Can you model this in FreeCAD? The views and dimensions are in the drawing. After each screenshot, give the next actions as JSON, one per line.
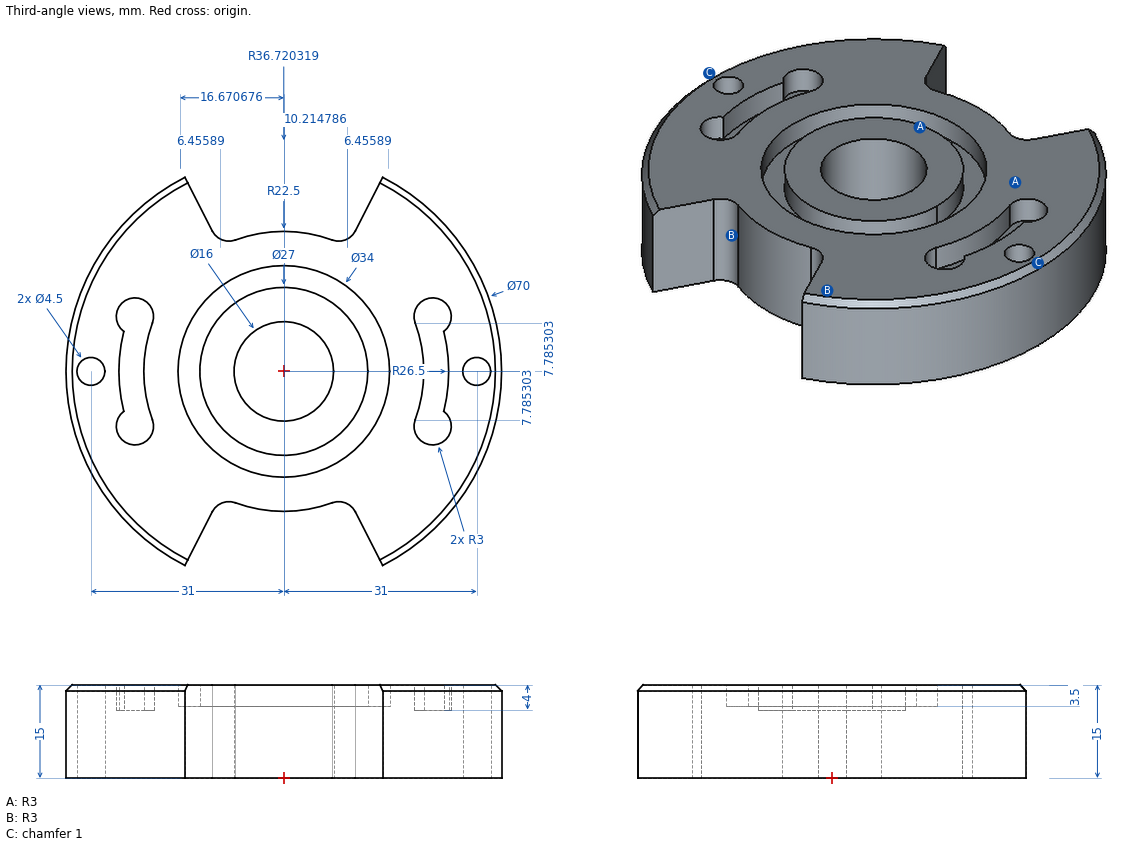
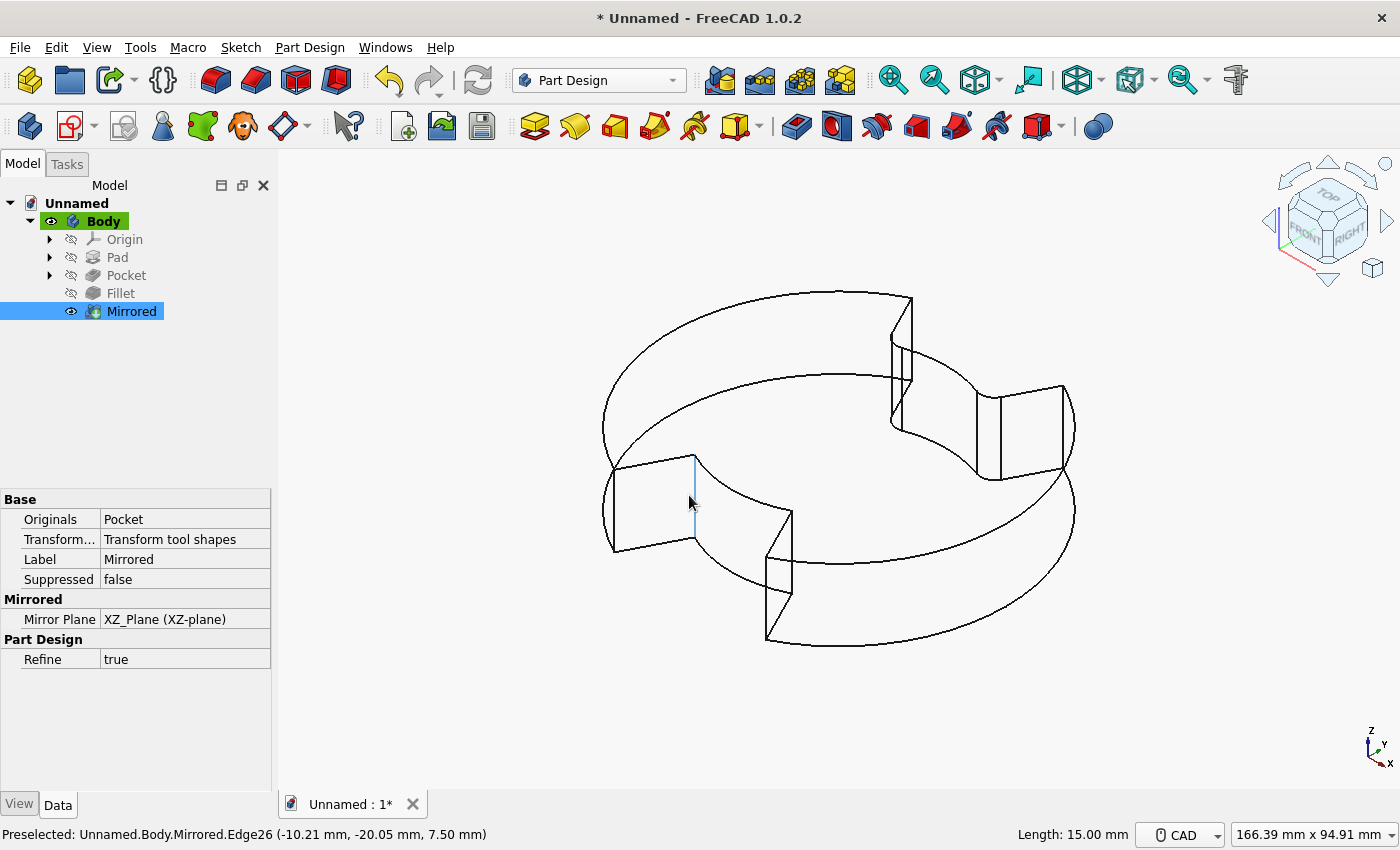
{"action": "left_click", "coordinate": [792, 551], "text": "ctrl"}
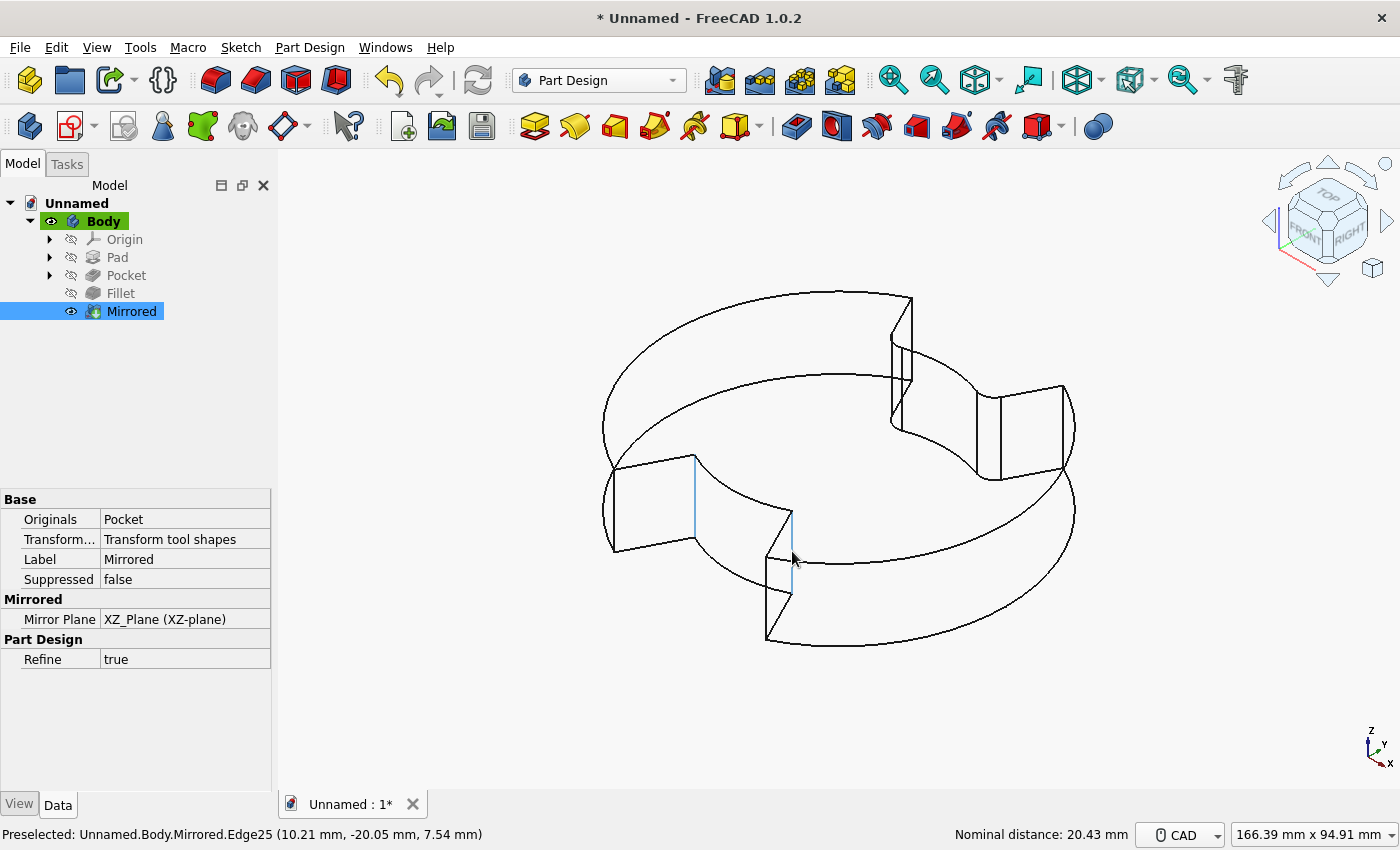
{"action": "key", "text": "v 1"}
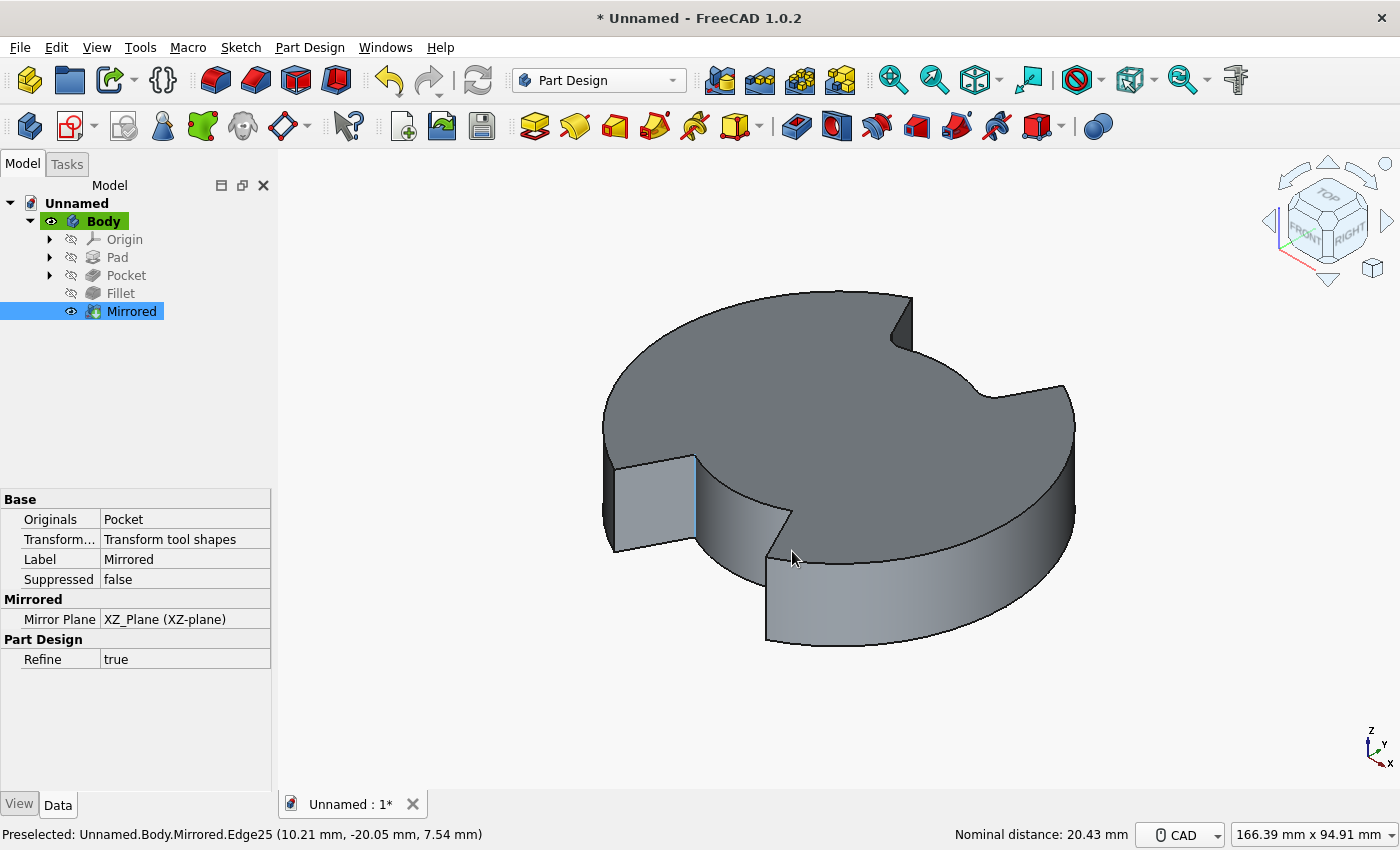
{"action": "left_click", "coordinate": [216, 80]}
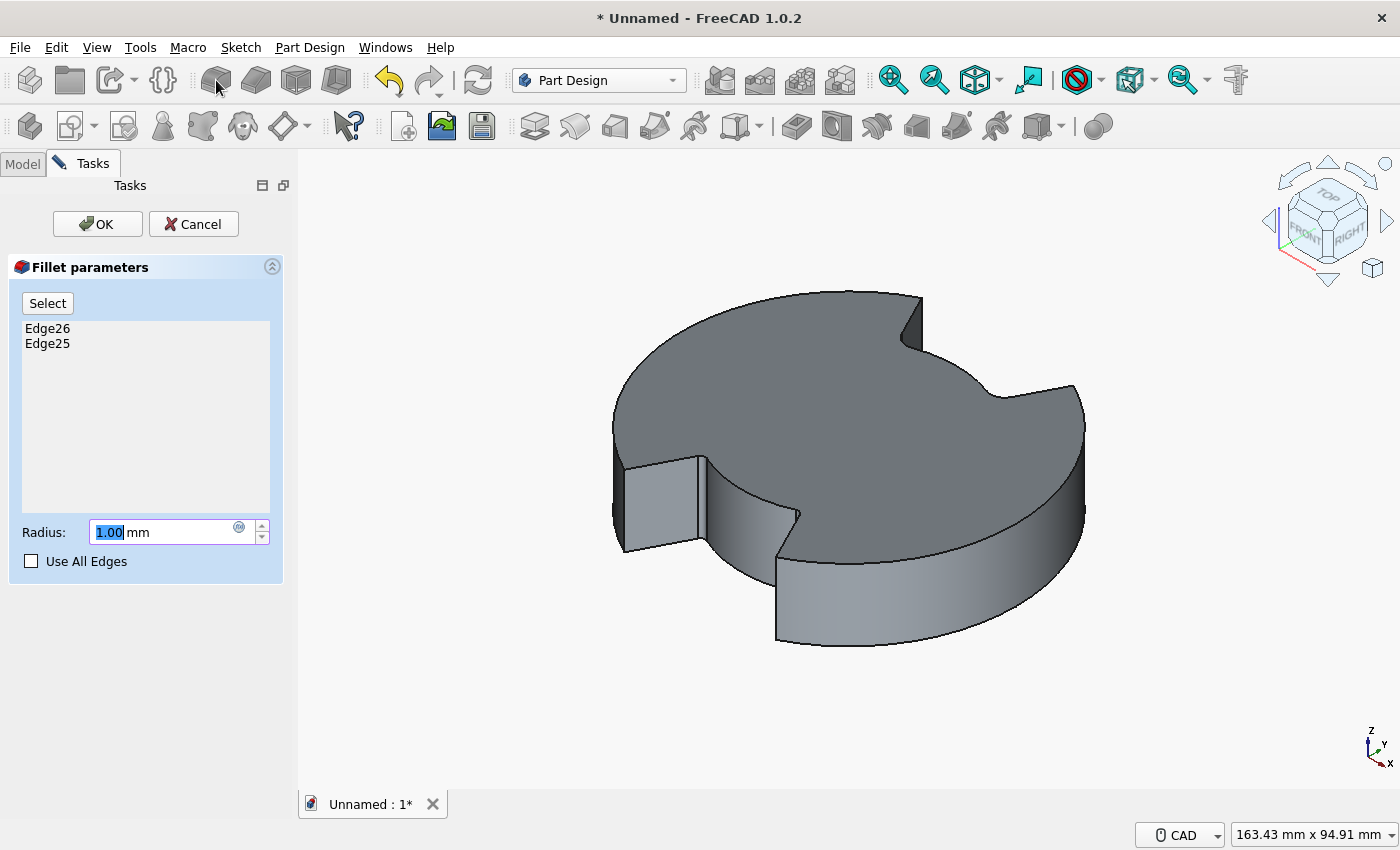
{"action": "type", "text": "3"}
{"action": "key", "text": "Tab"}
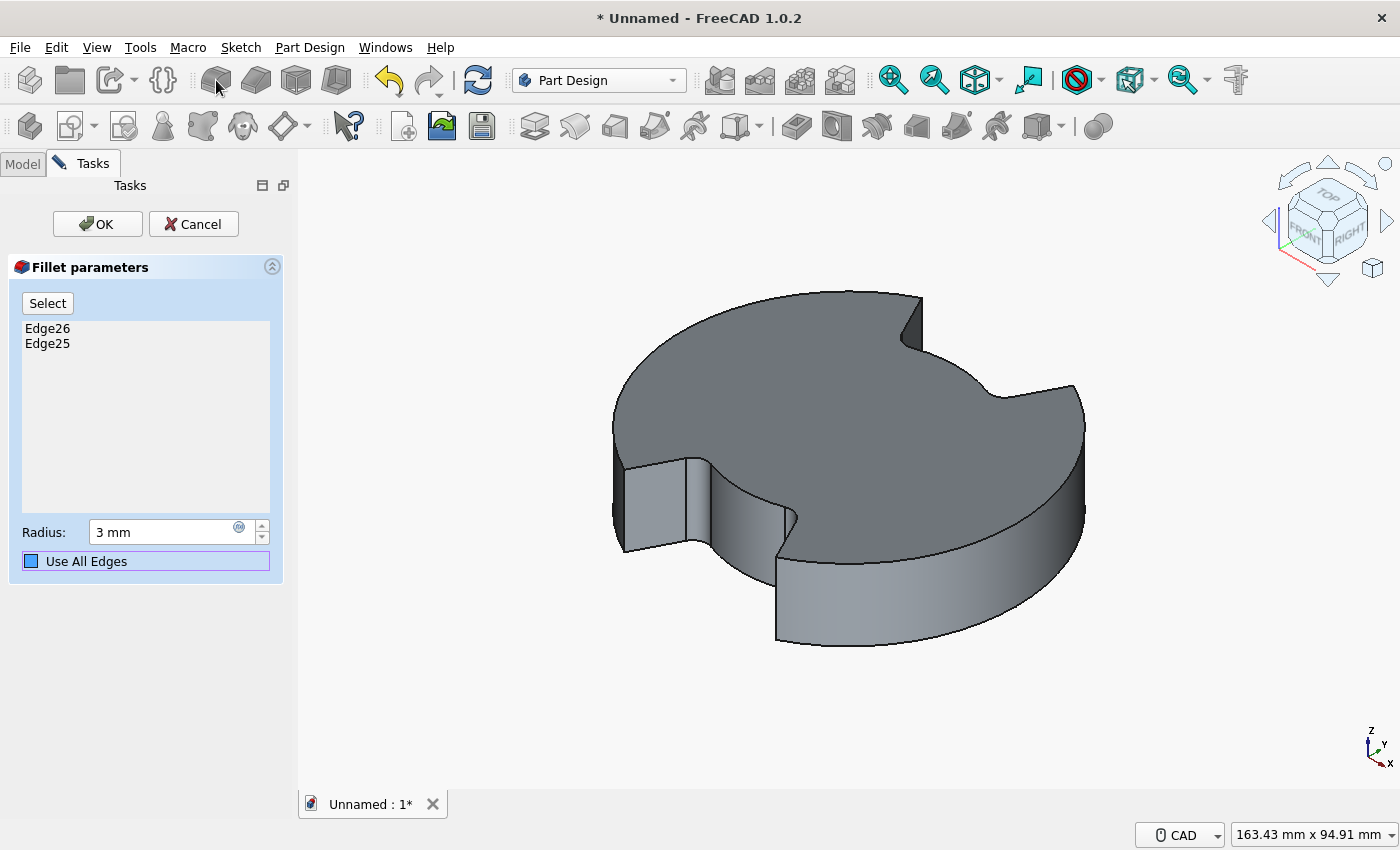
{"action": "left_click", "coordinate": [98, 224]}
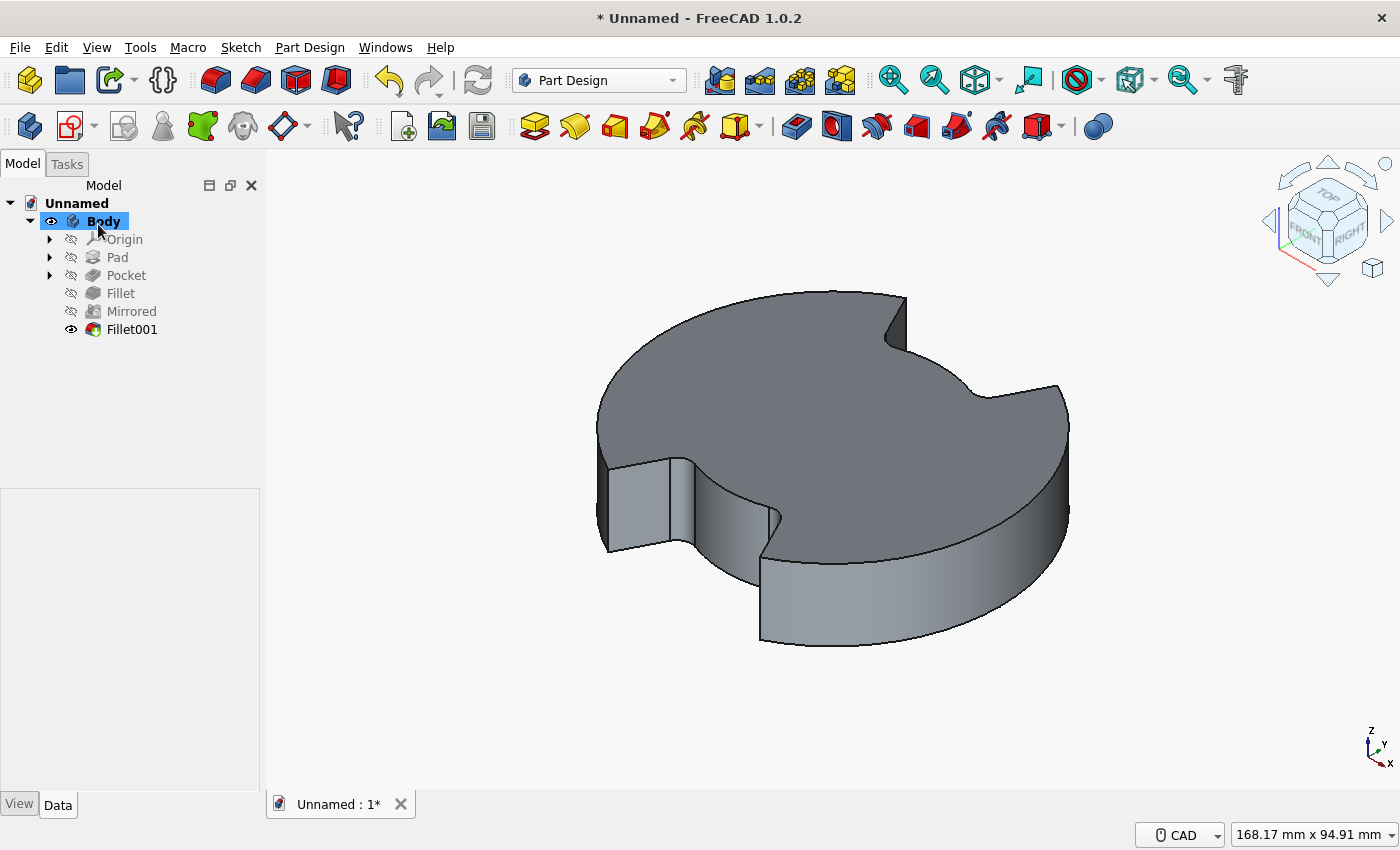
{"action": "left_click", "coordinate": [833, 427]}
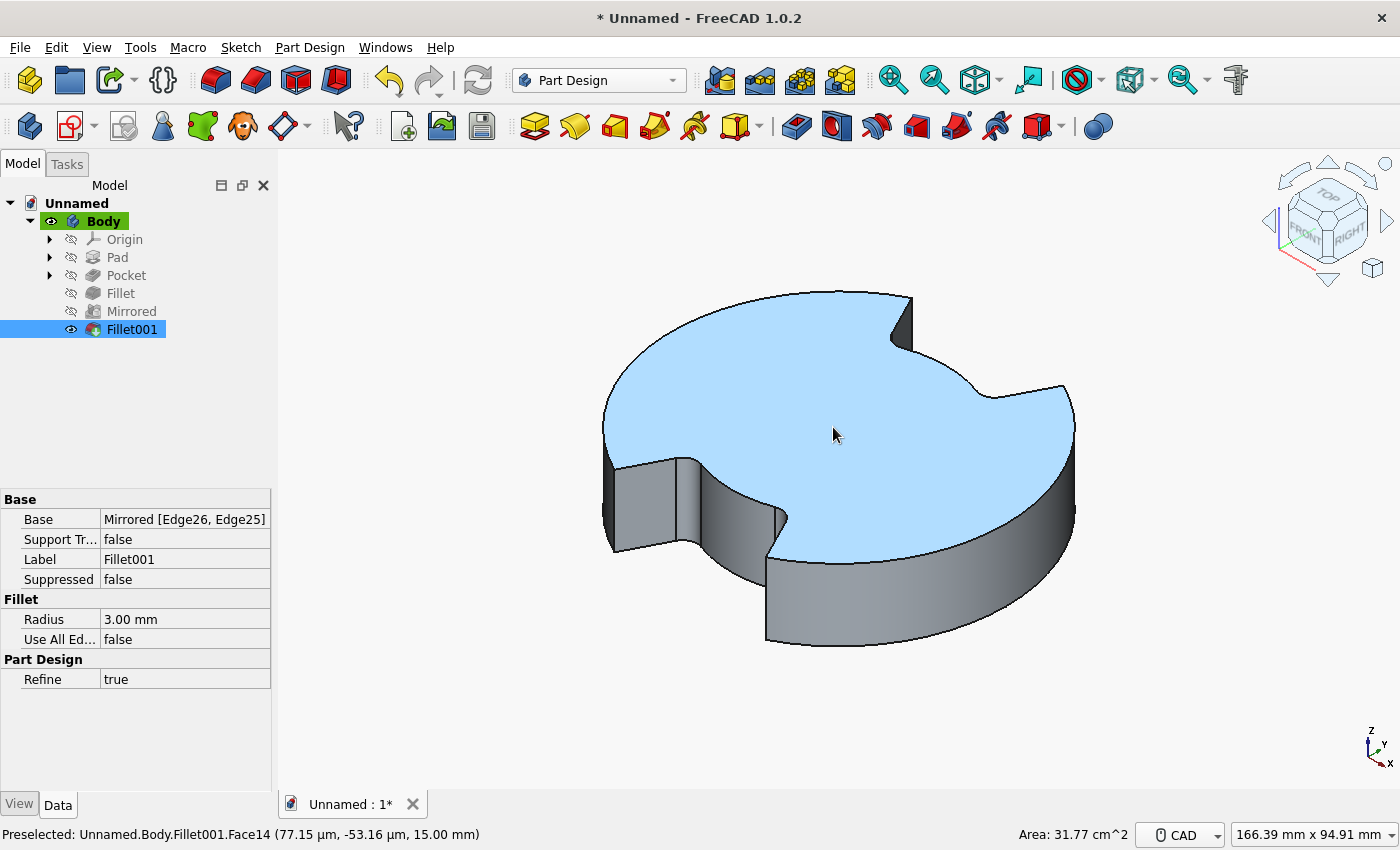
{"action": "left_click", "coordinate": [70, 126]}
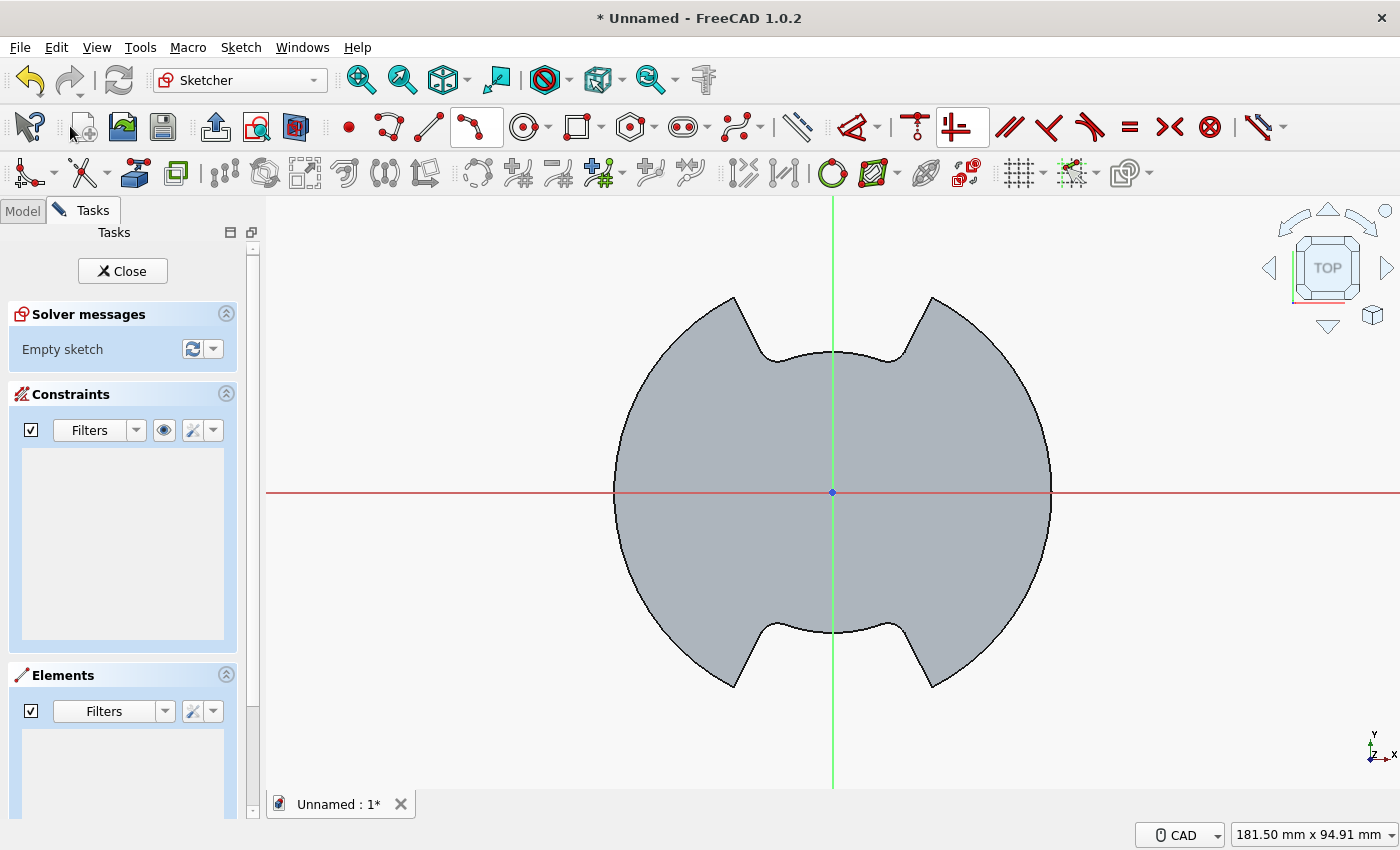
{"action": "scroll", "coordinate": [916, 493], "scroll_direction": "up", "scroll_amount": 3}